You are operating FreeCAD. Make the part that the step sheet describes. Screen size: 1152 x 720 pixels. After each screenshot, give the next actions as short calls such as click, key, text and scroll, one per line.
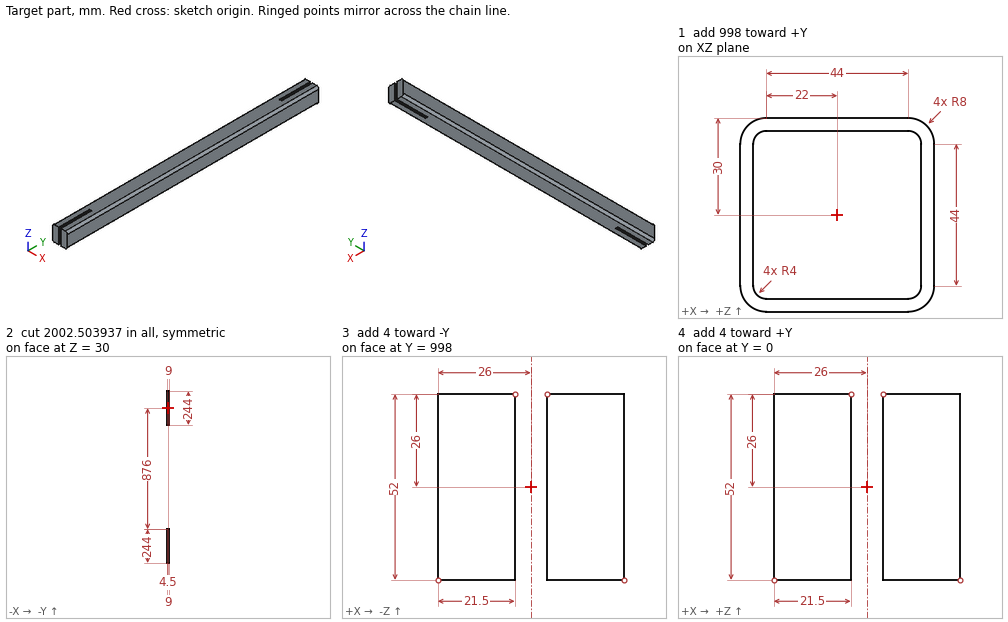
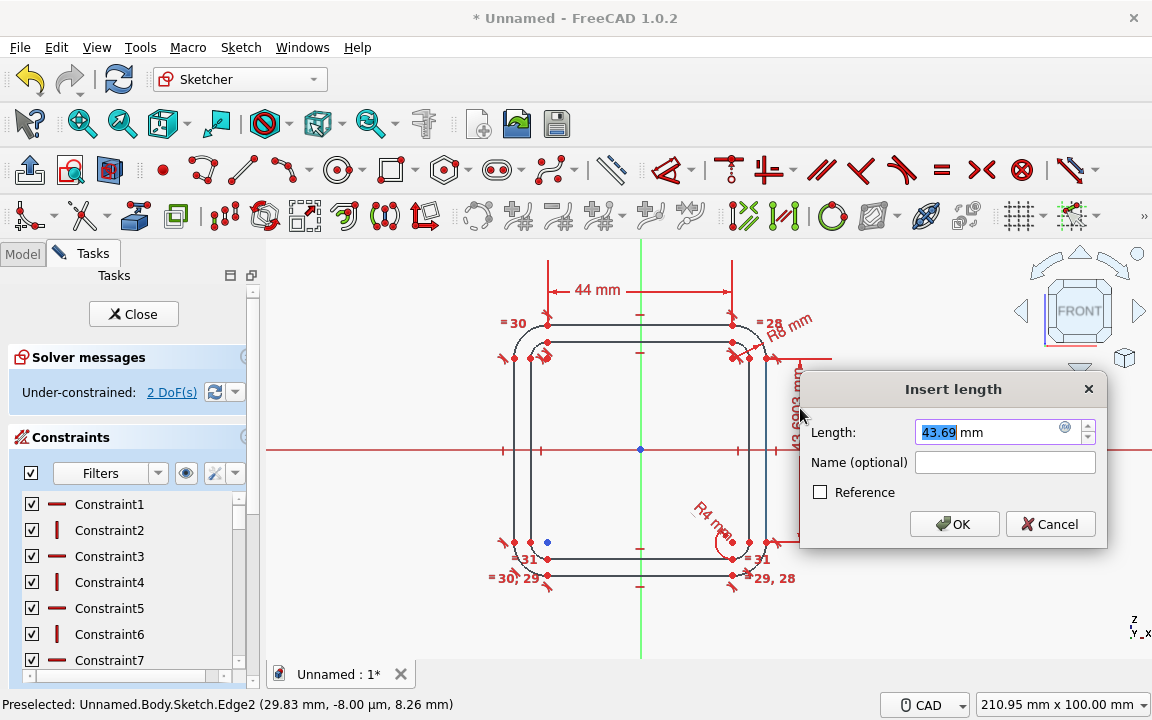
text(44)
key(Return)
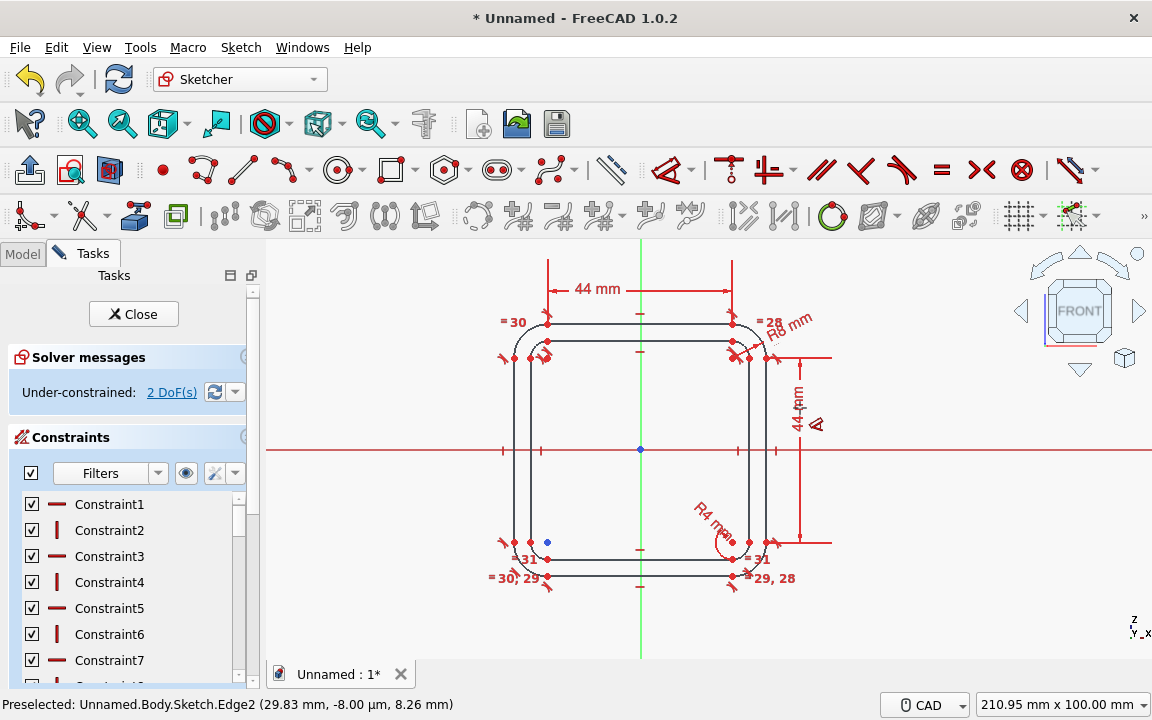
click(548, 324)
click(594, 484)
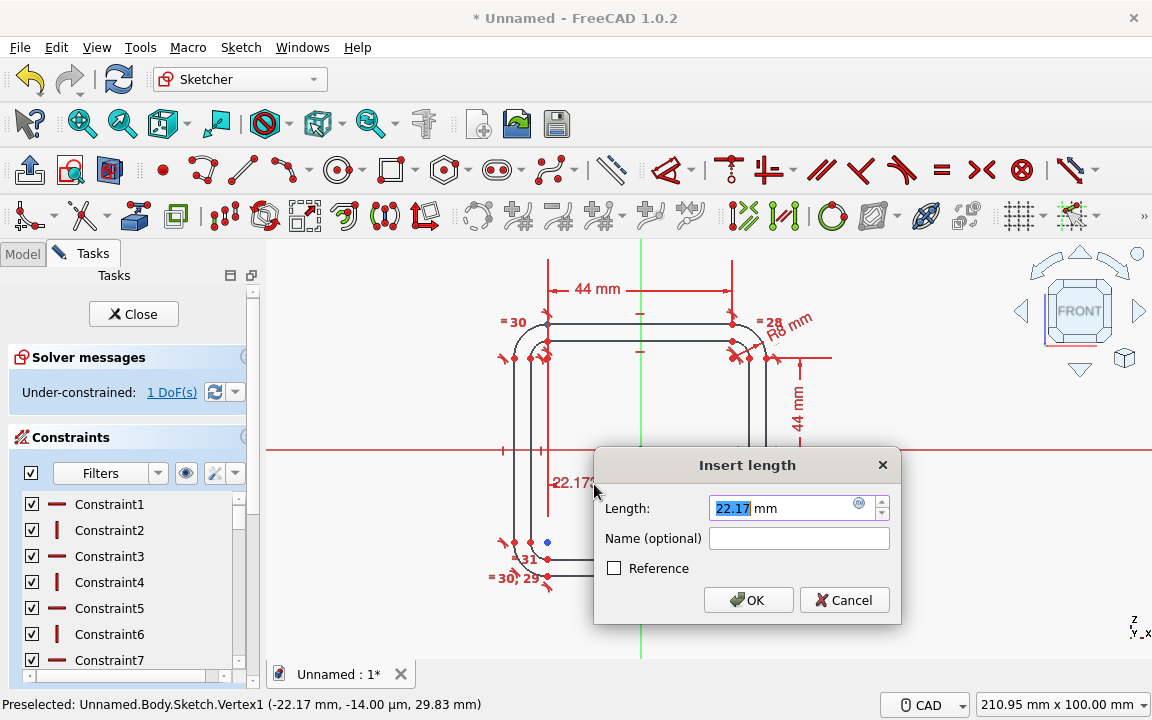
text(22)
key(Return)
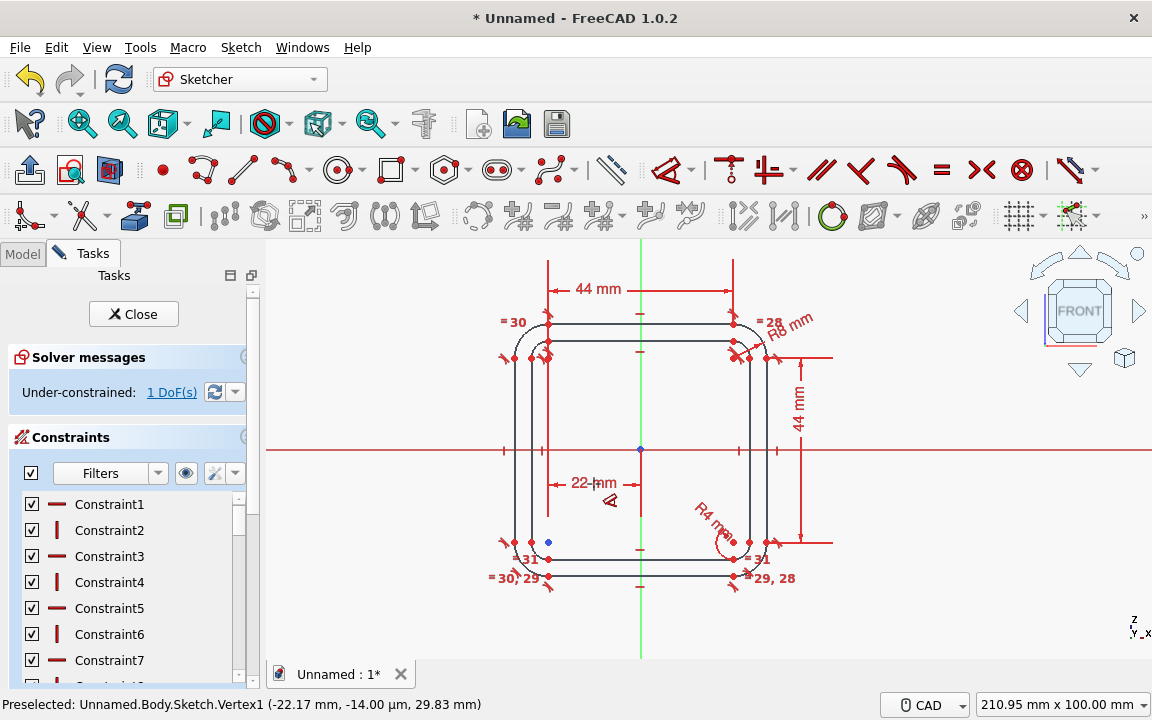
click(548, 324)
click(675, 387)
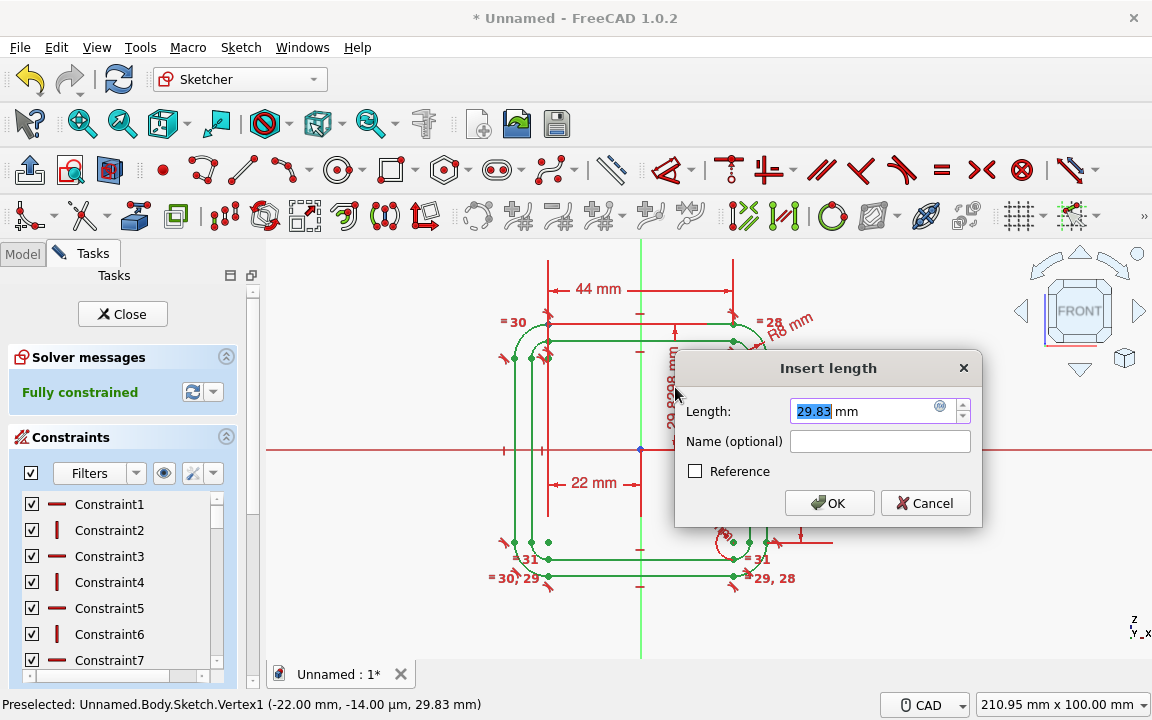
text(30)
key(Return)
key(Escape)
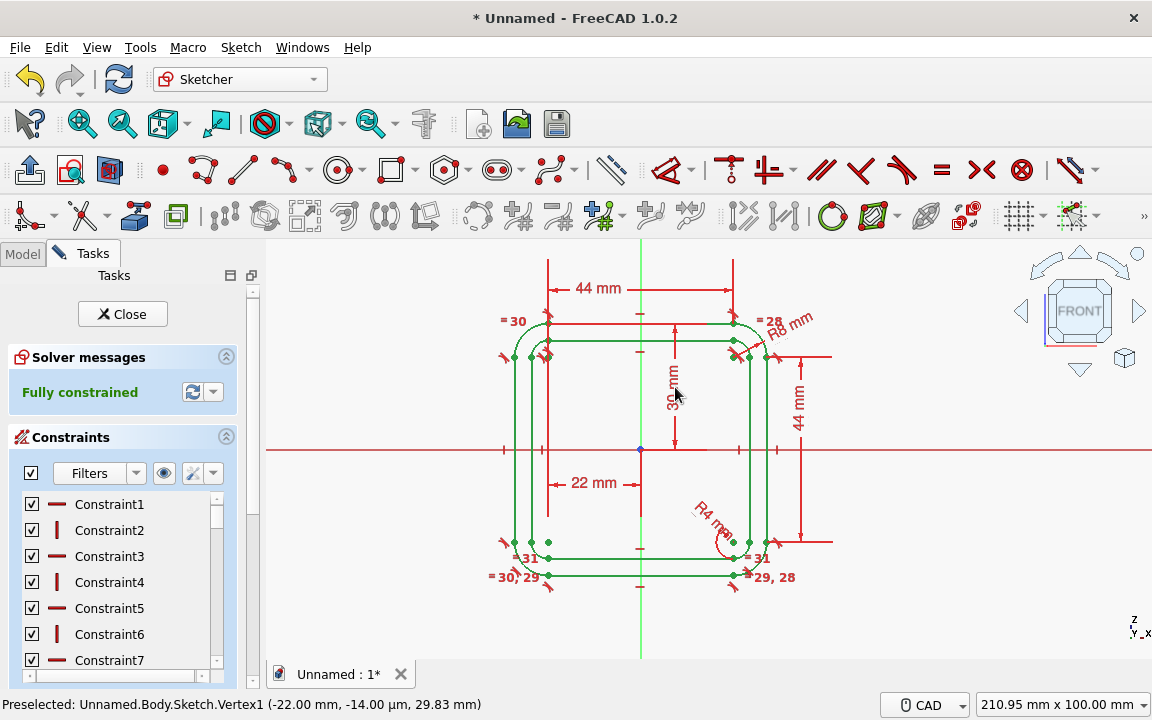
click(123, 314)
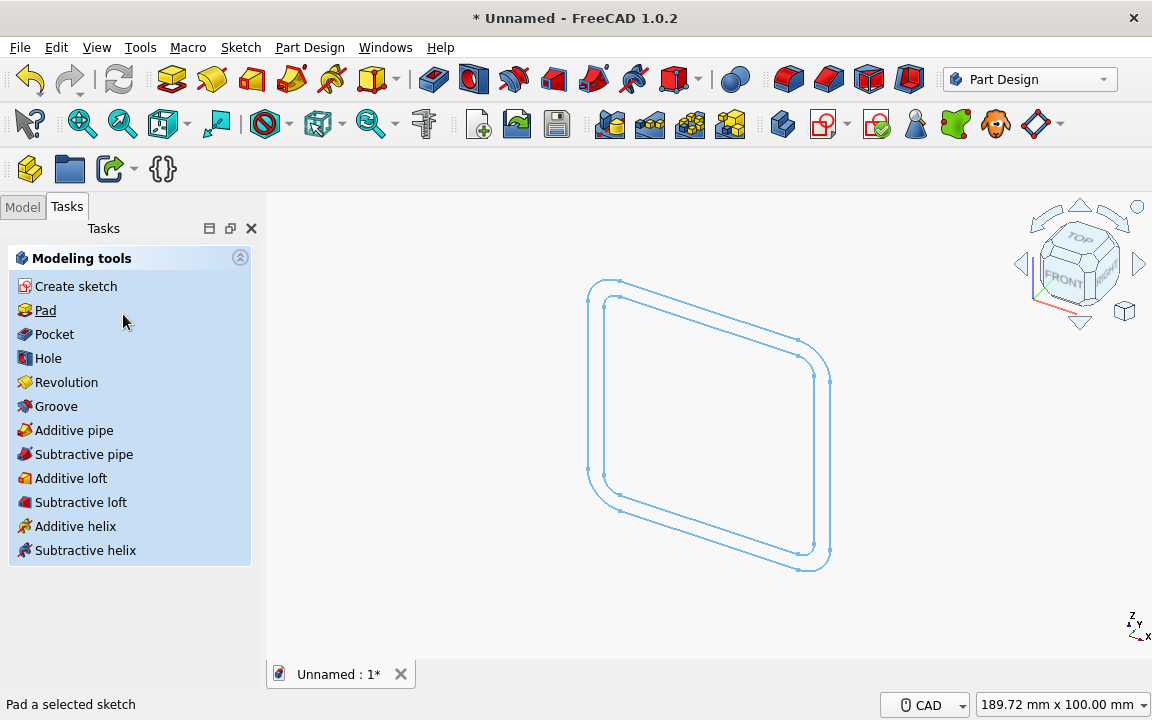
click(172, 80)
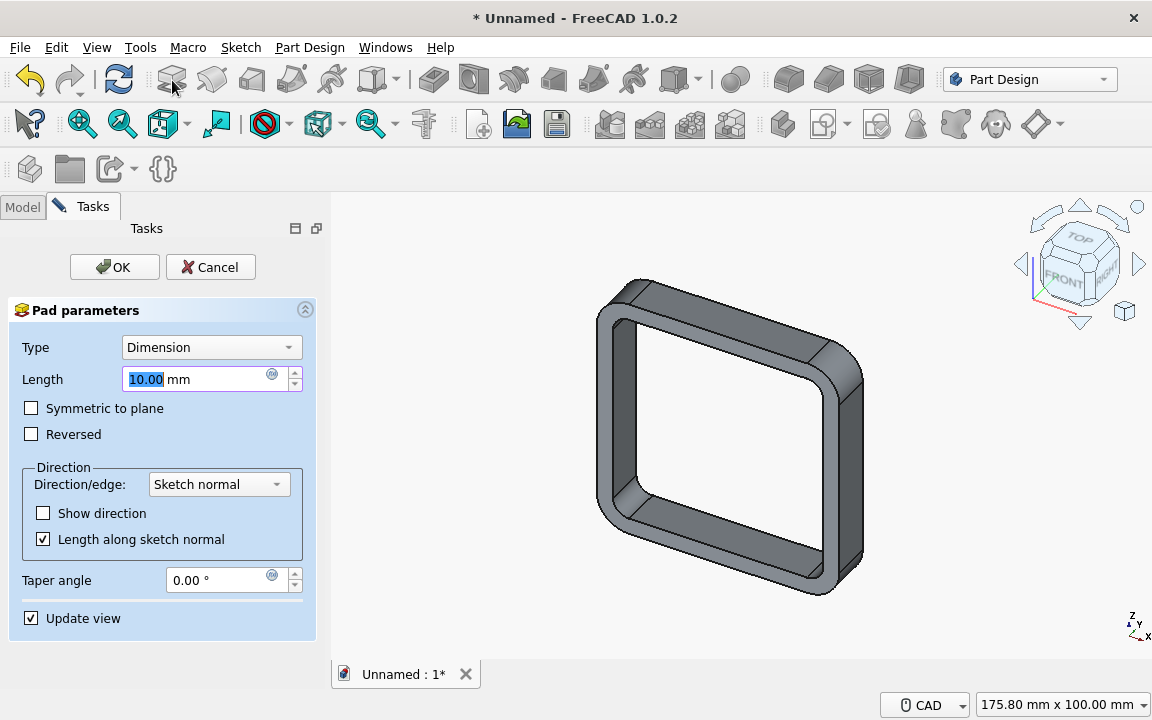
text(998)
key(Tab)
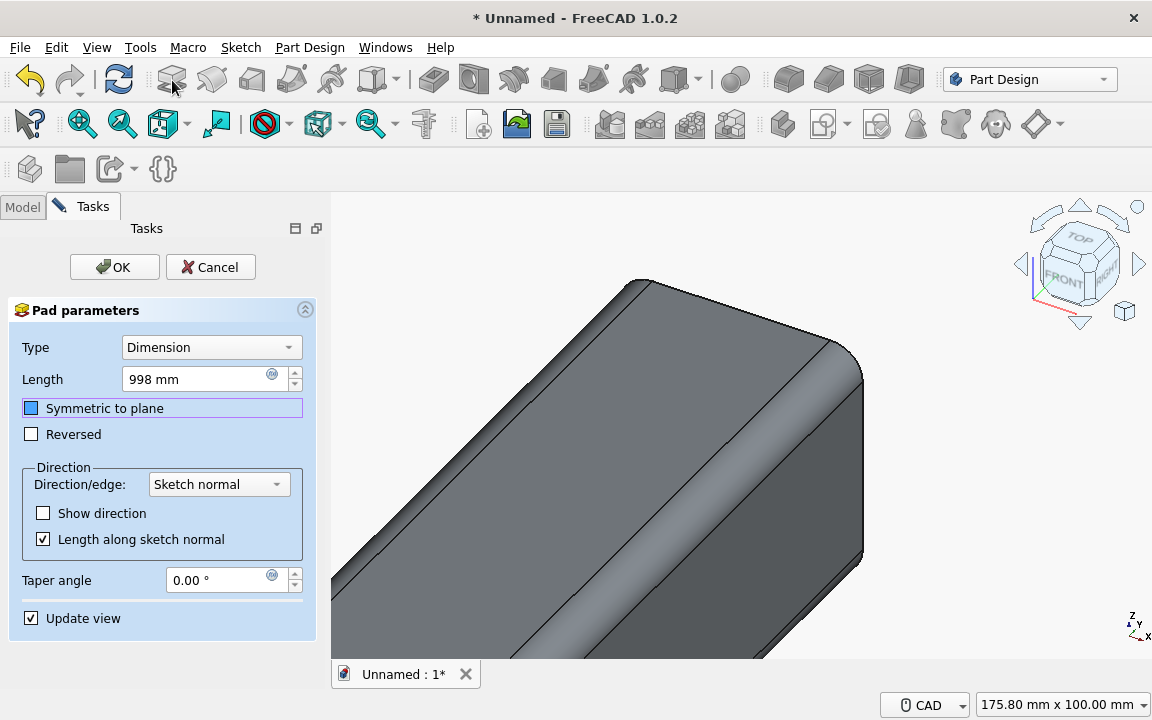
click(30, 434)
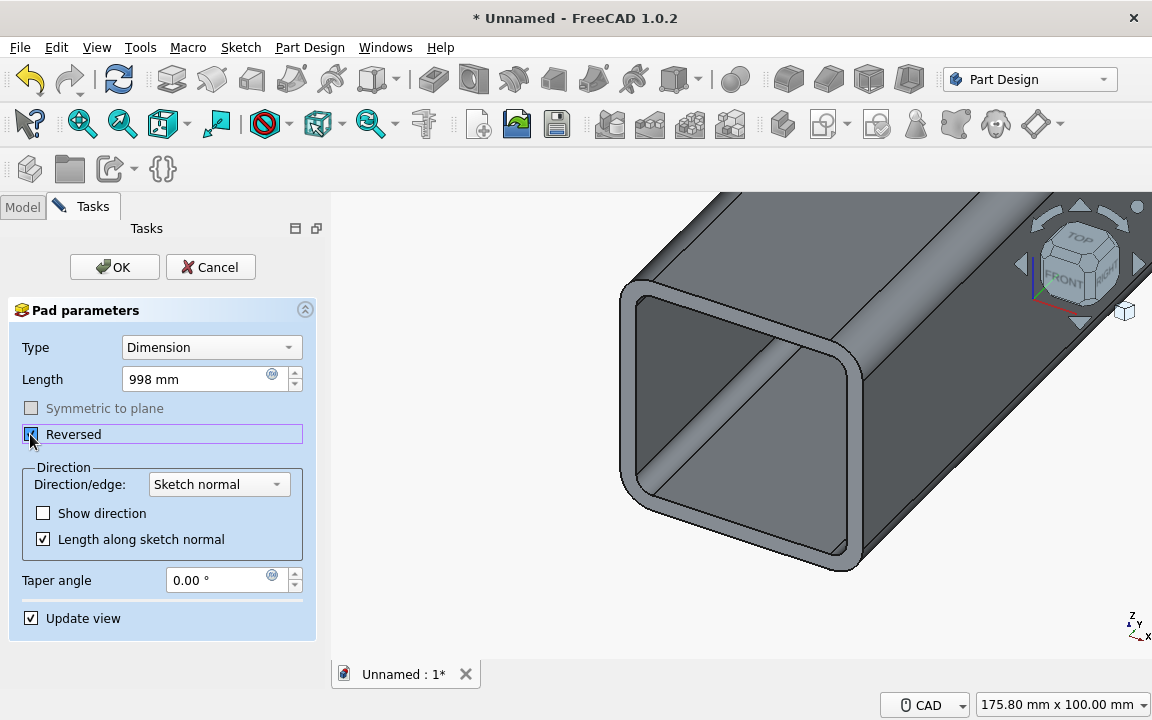
click(115, 267)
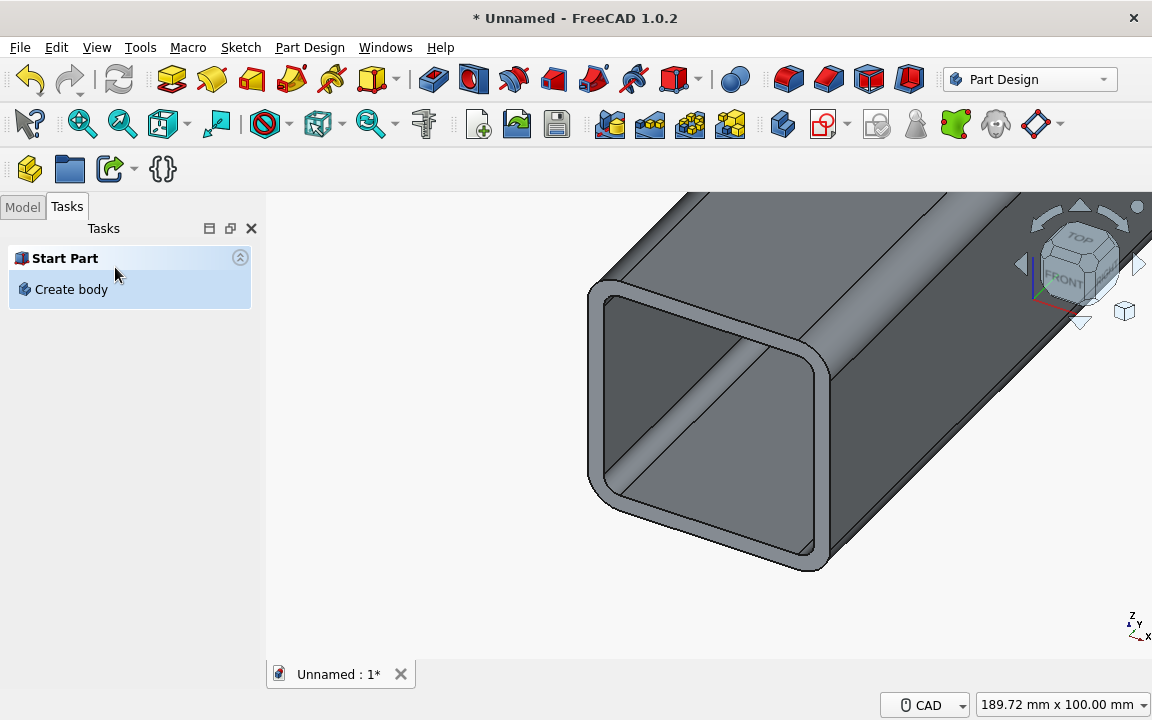
click(84, 124)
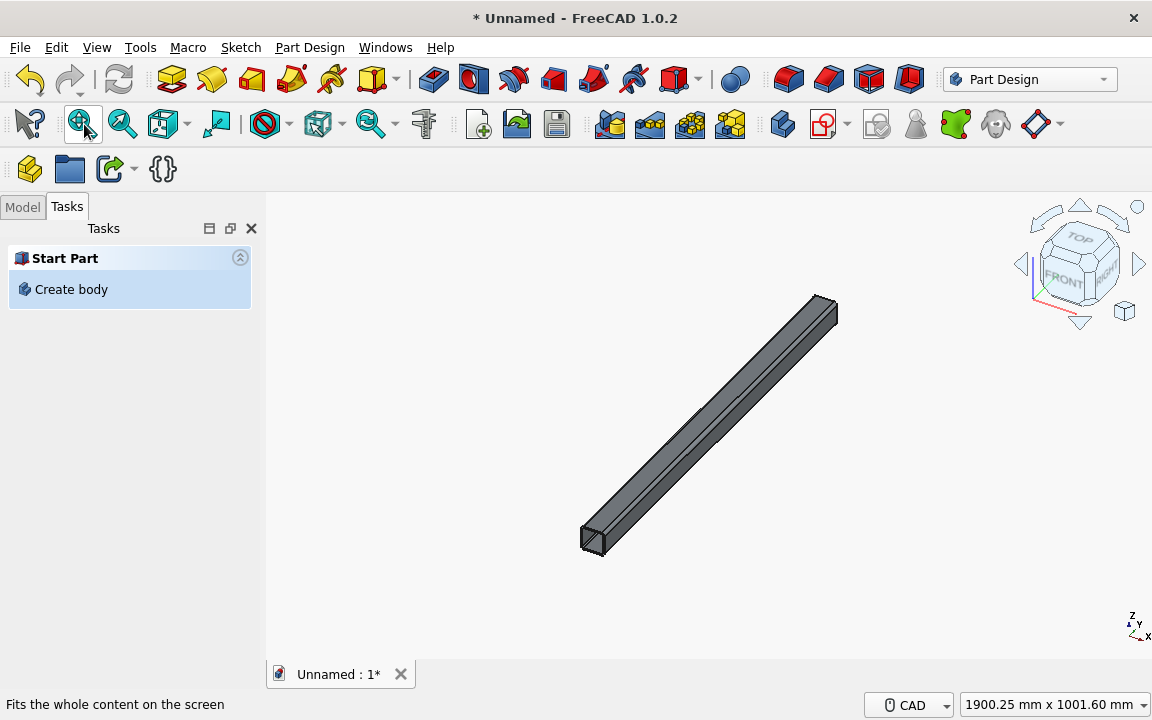
key(0)